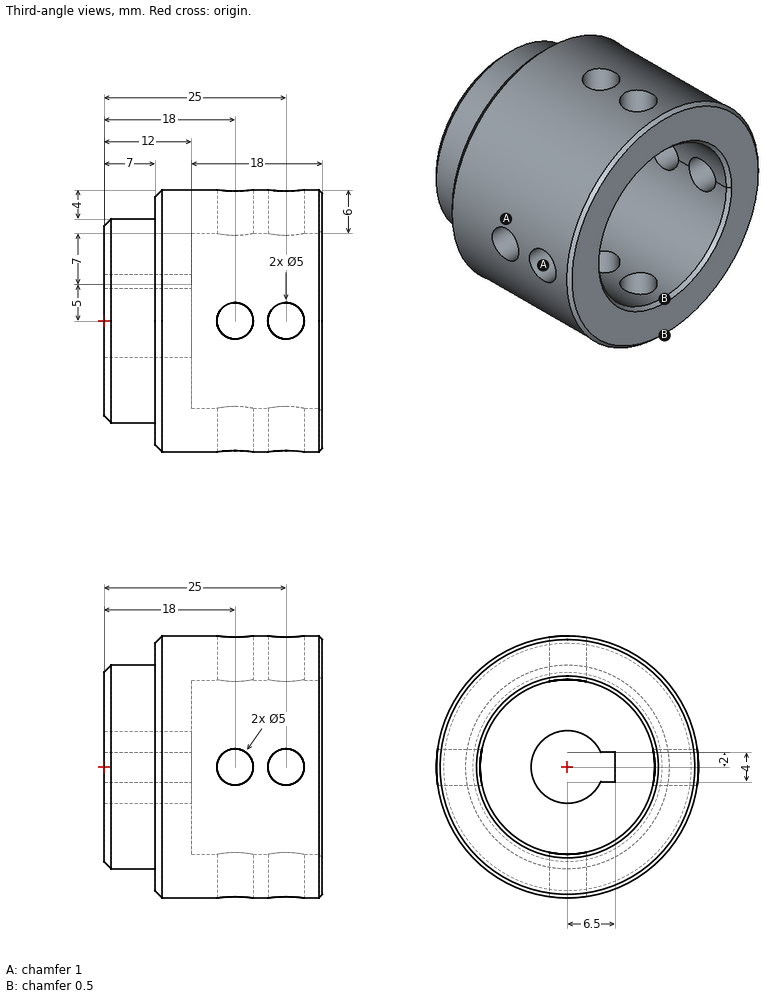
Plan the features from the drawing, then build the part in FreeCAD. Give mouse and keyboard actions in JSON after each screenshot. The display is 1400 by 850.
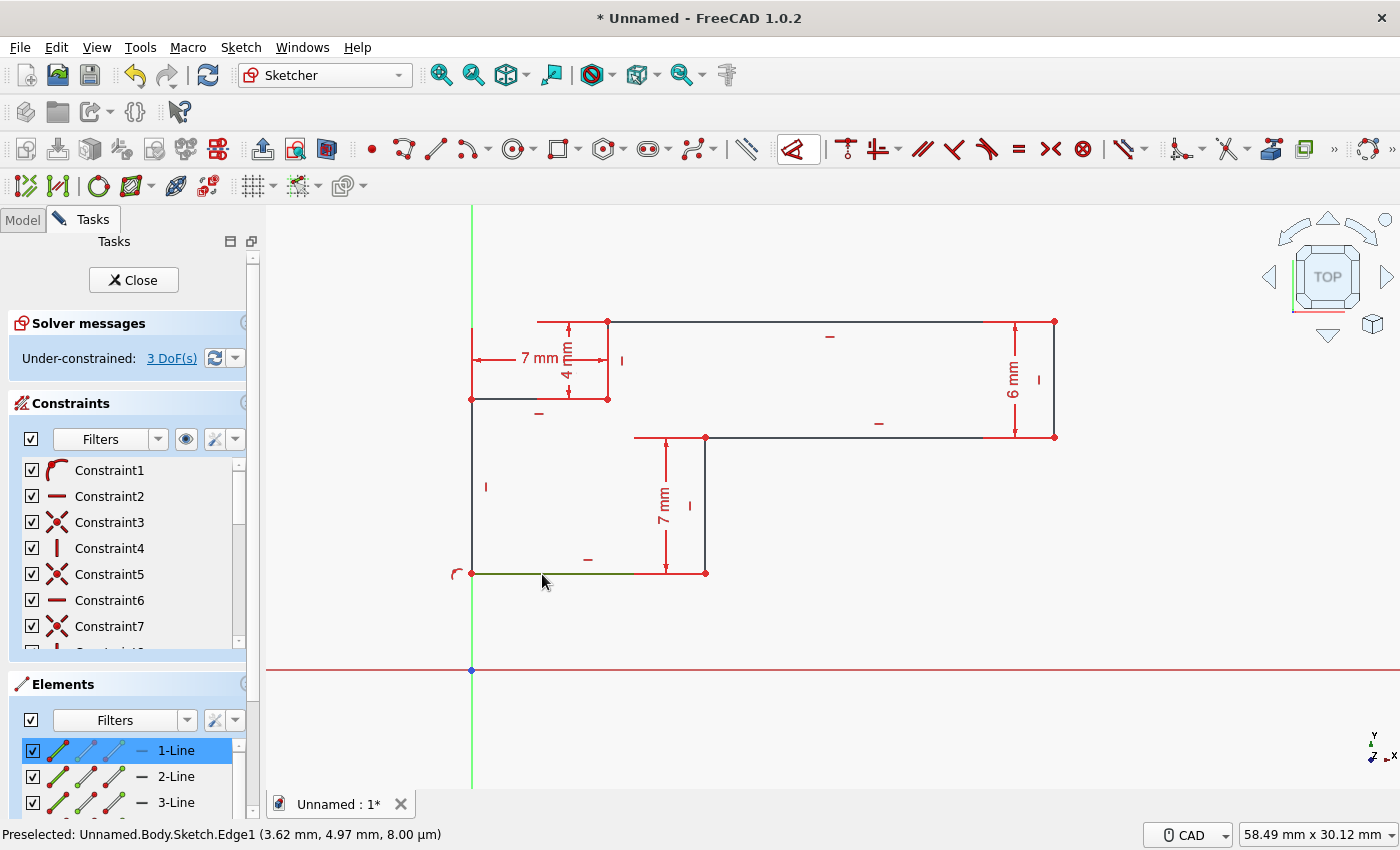
{"action": "left_click", "coordinate": [814, 150]}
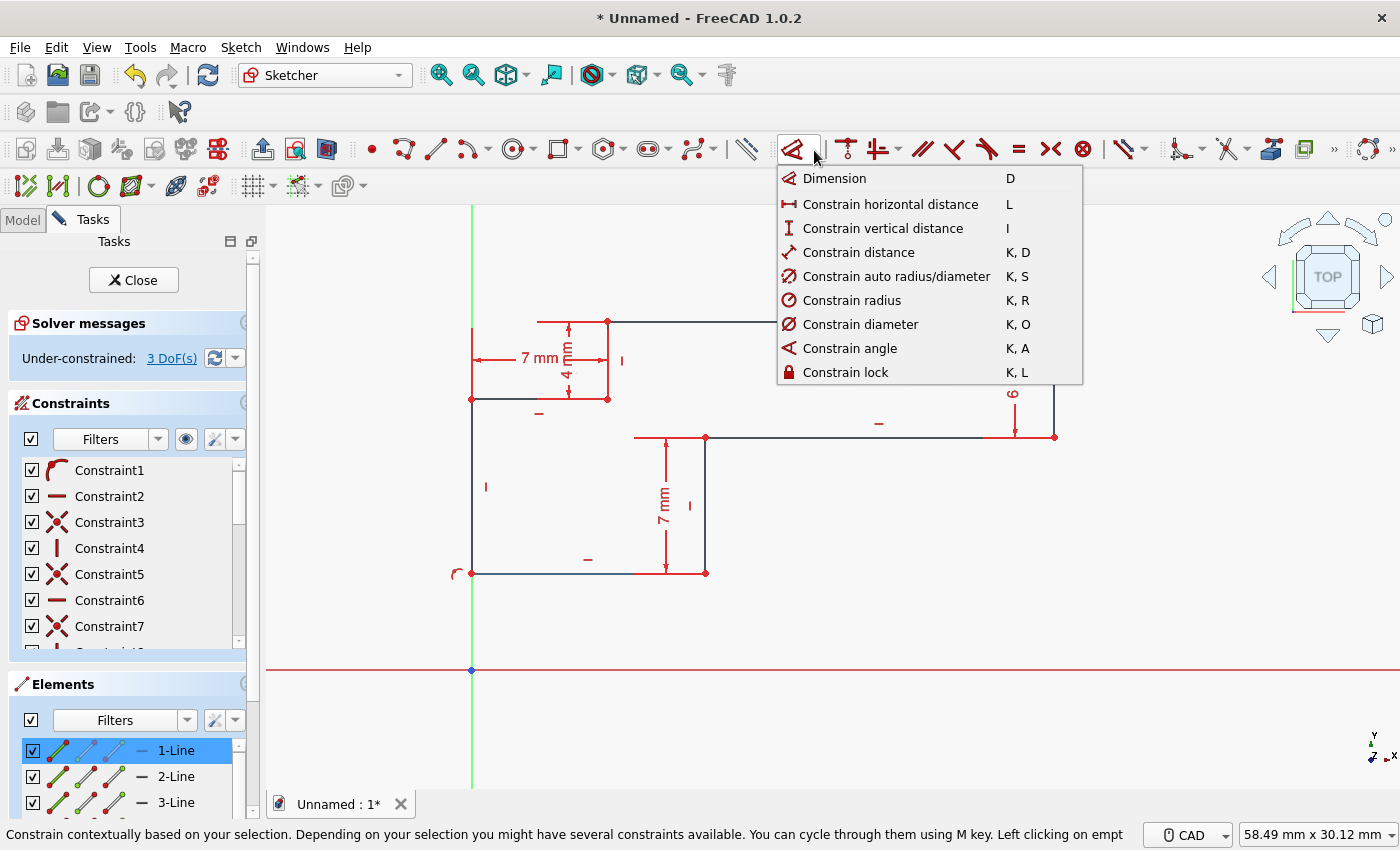
{"action": "left_click", "coordinate": [930, 204]}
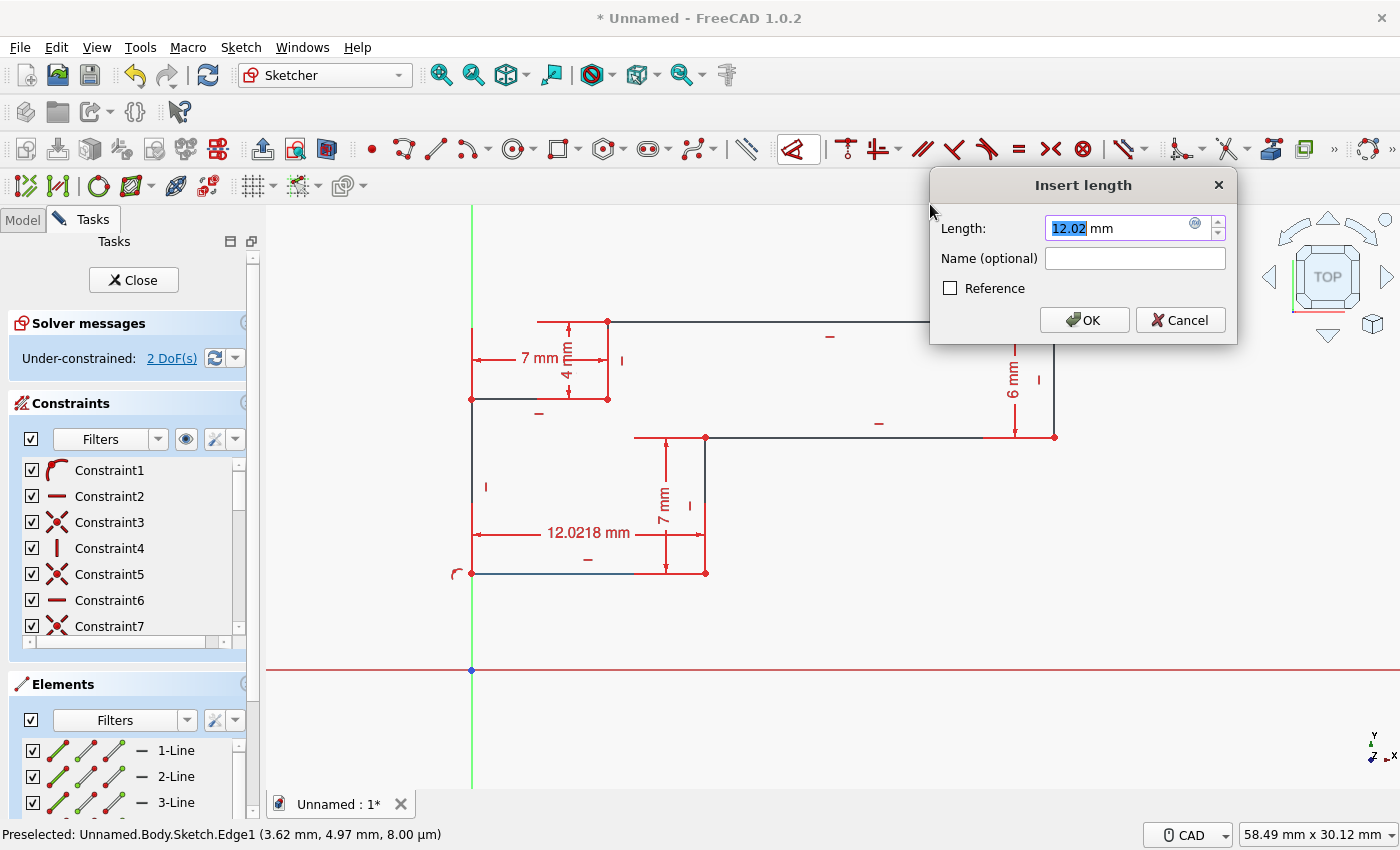
{"action": "type", "text": "12"}
{"action": "key", "text": "Return"}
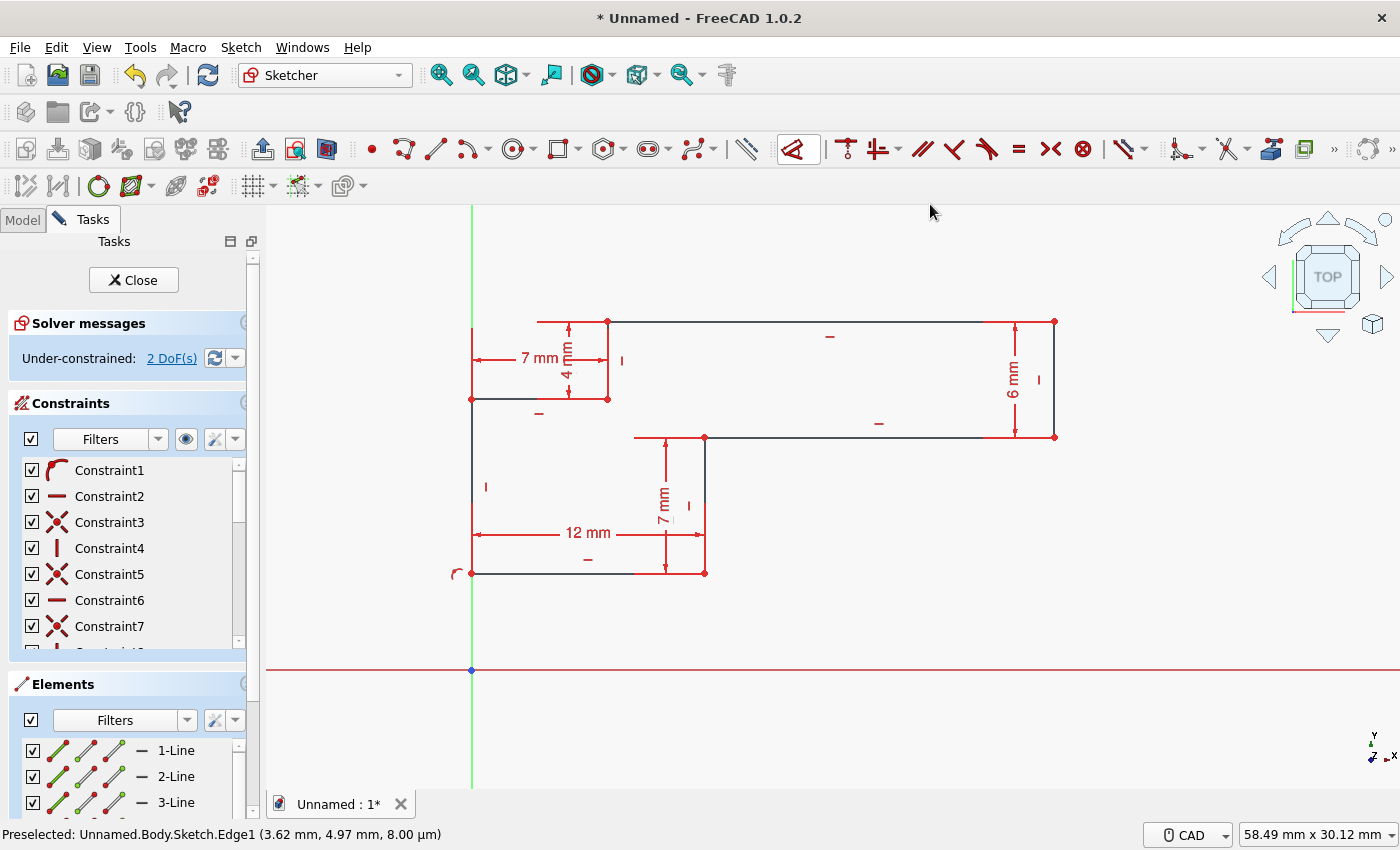
{"action": "left_click", "coordinate": [809, 438]}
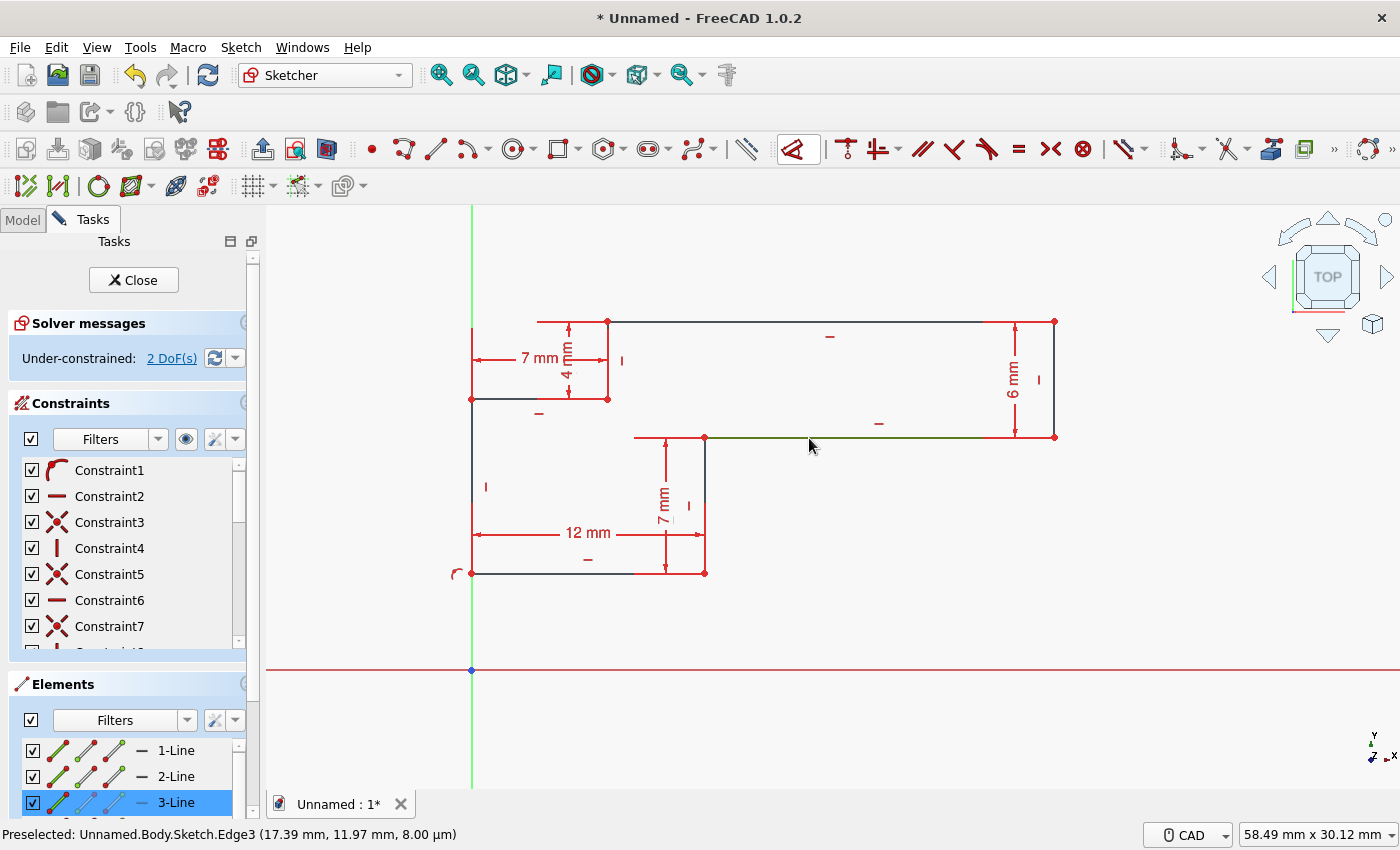
{"action": "left_click", "coordinate": [814, 150]}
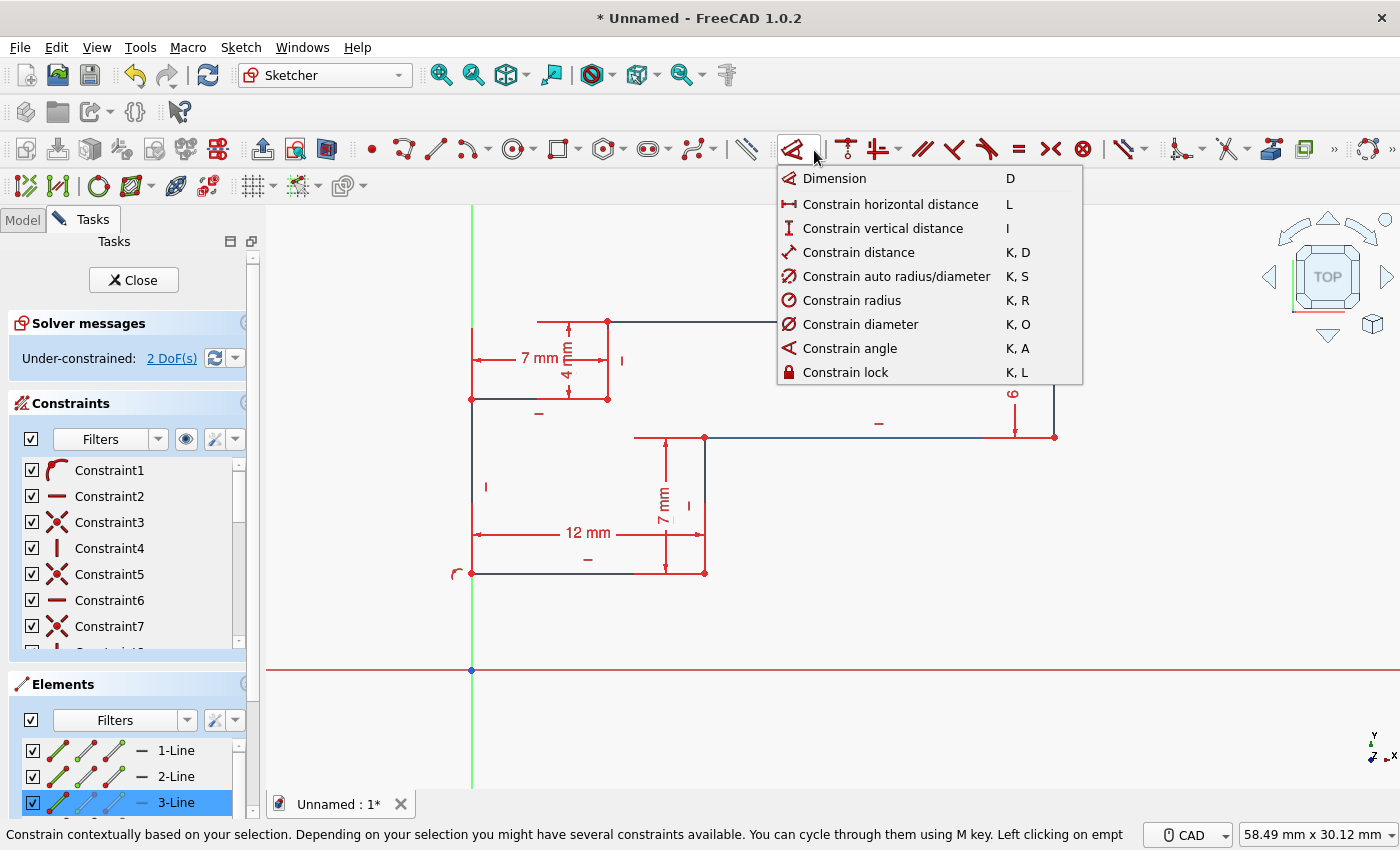
{"action": "left_click", "coordinate": [930, 204]}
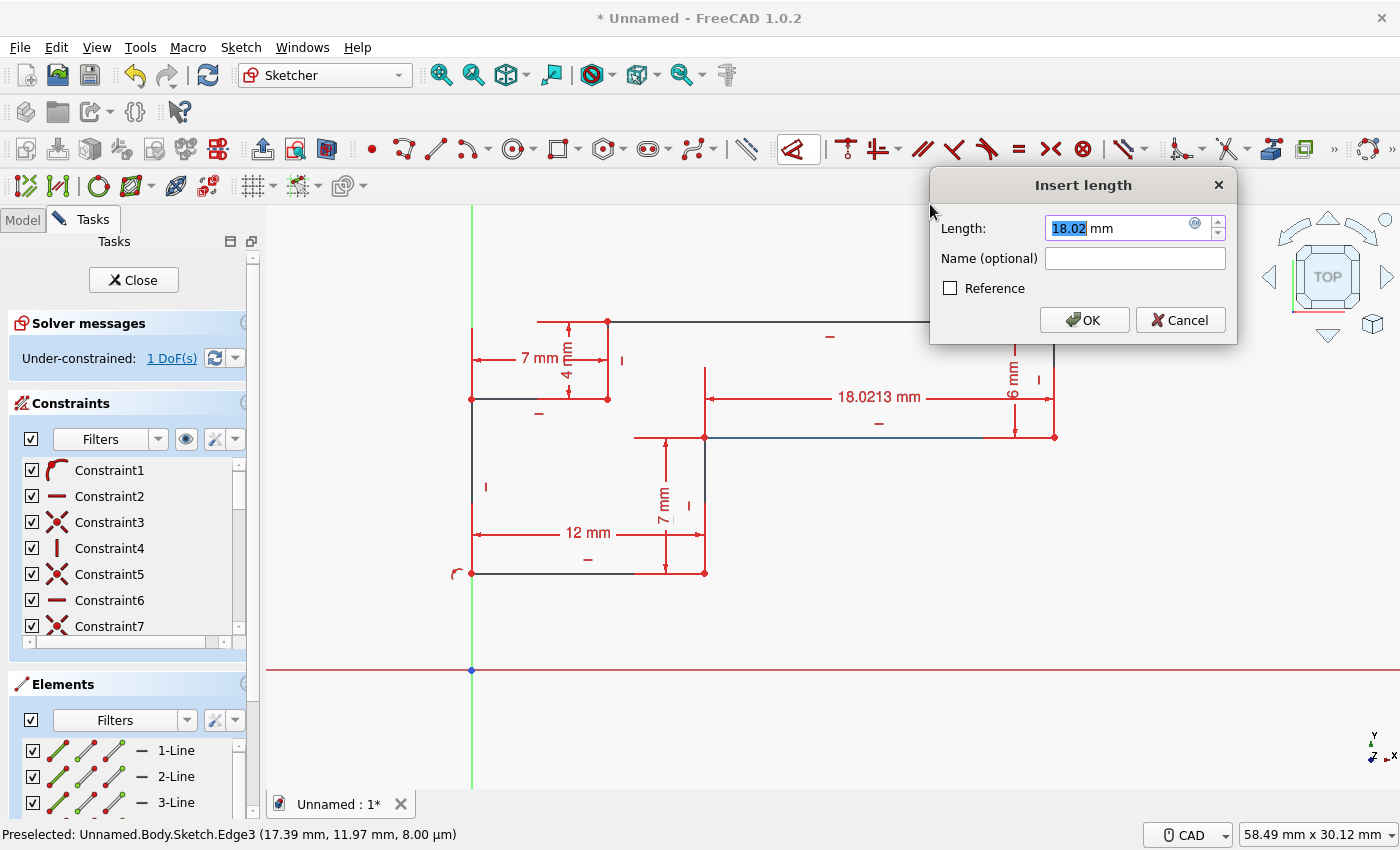
{"action": "type", "text": "18"}
{"action": "key", "text": "Return"}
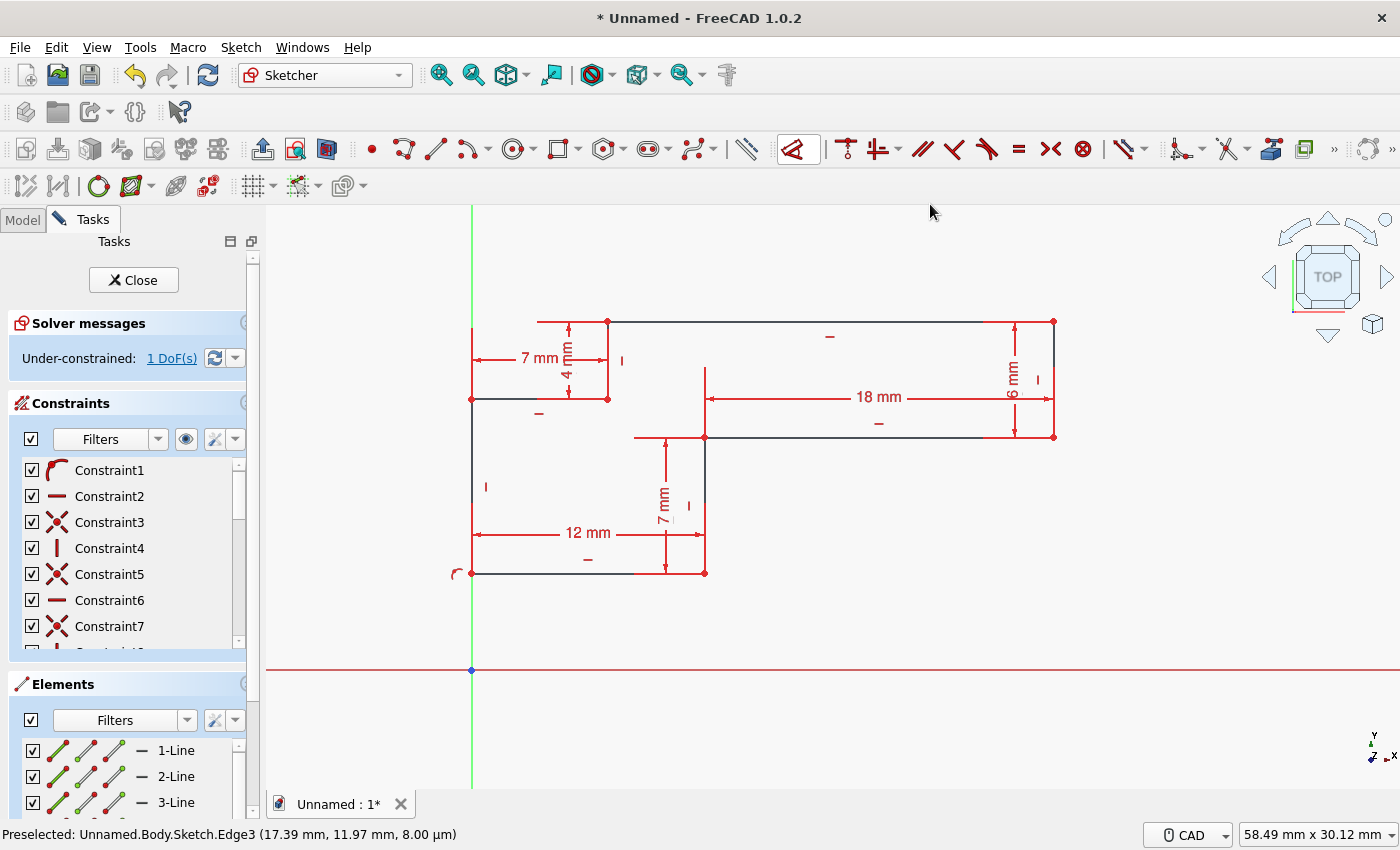
{"action": "left_click", "coordinate": [472, 574]}